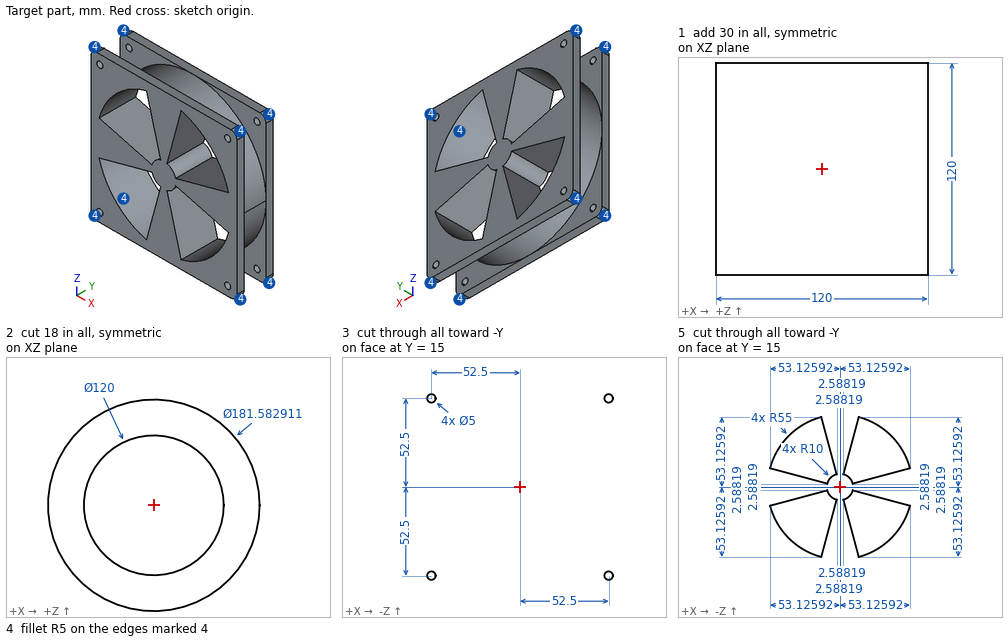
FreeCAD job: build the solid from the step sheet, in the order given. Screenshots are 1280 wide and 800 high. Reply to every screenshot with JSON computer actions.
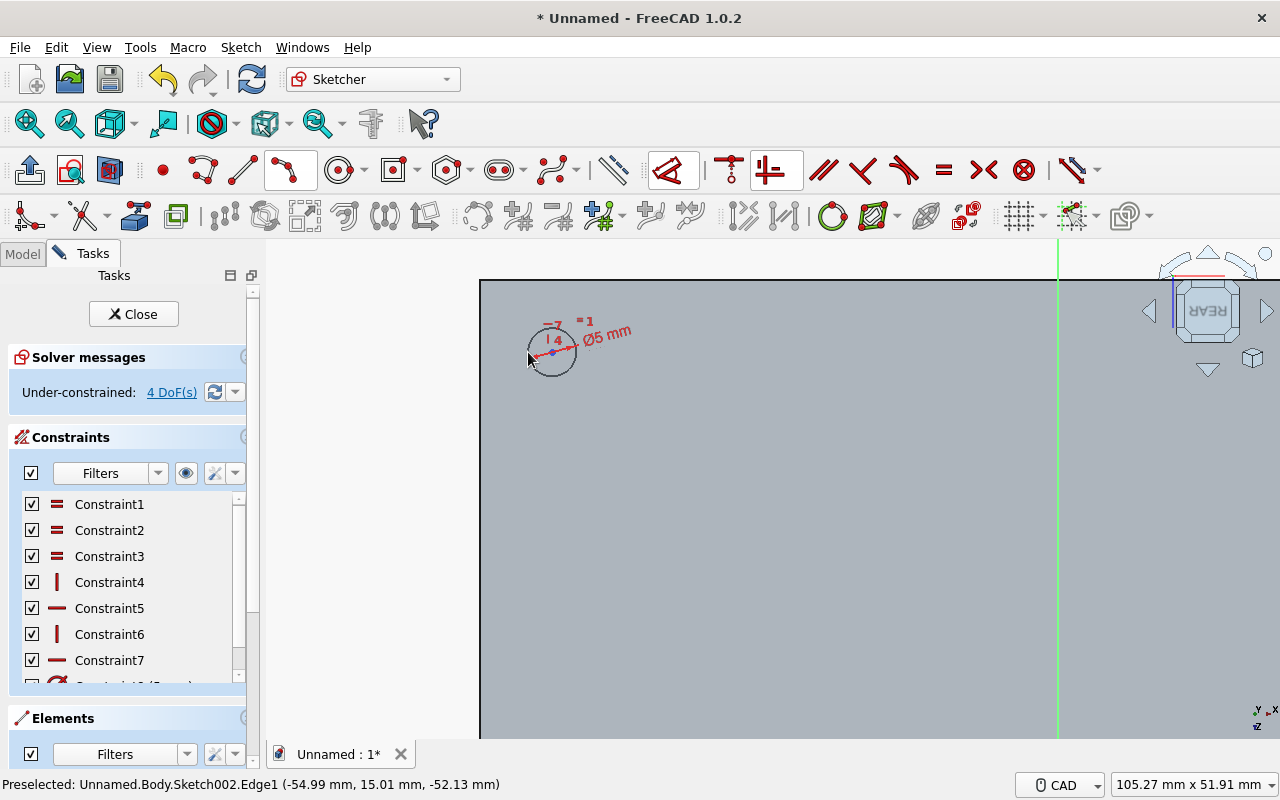
{"action": "left_click", "coordinate": [552, 352]}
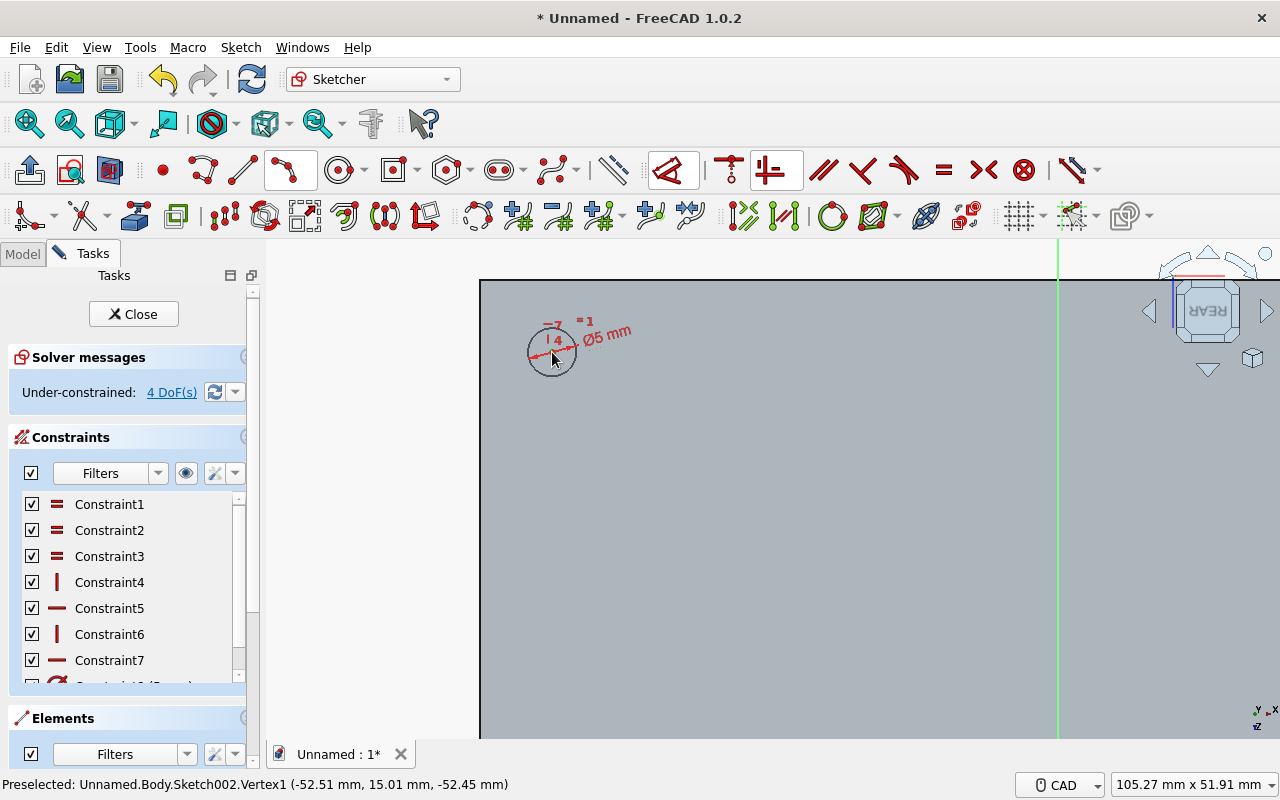
{"action": "key", "text": "l"}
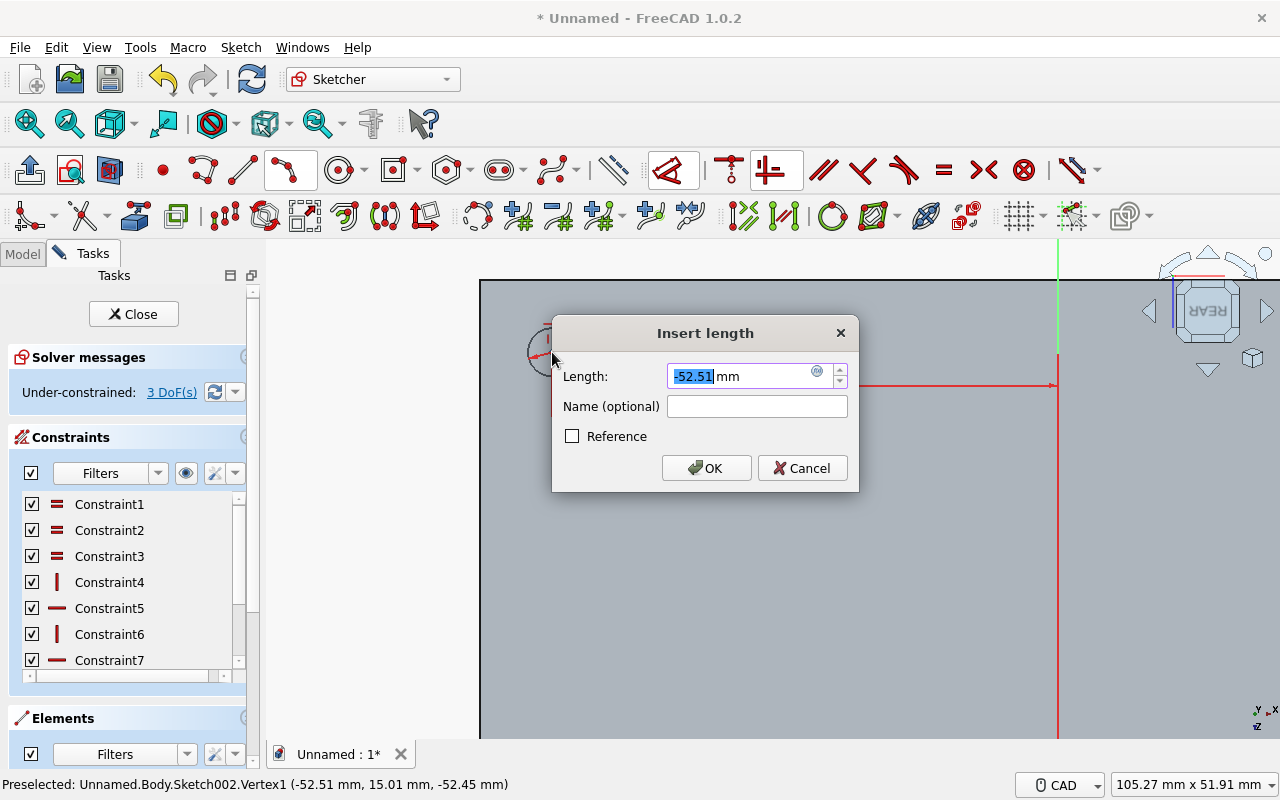
{"action": "type", "text": "-52.5"}
{"action": "key", "text": "Return"}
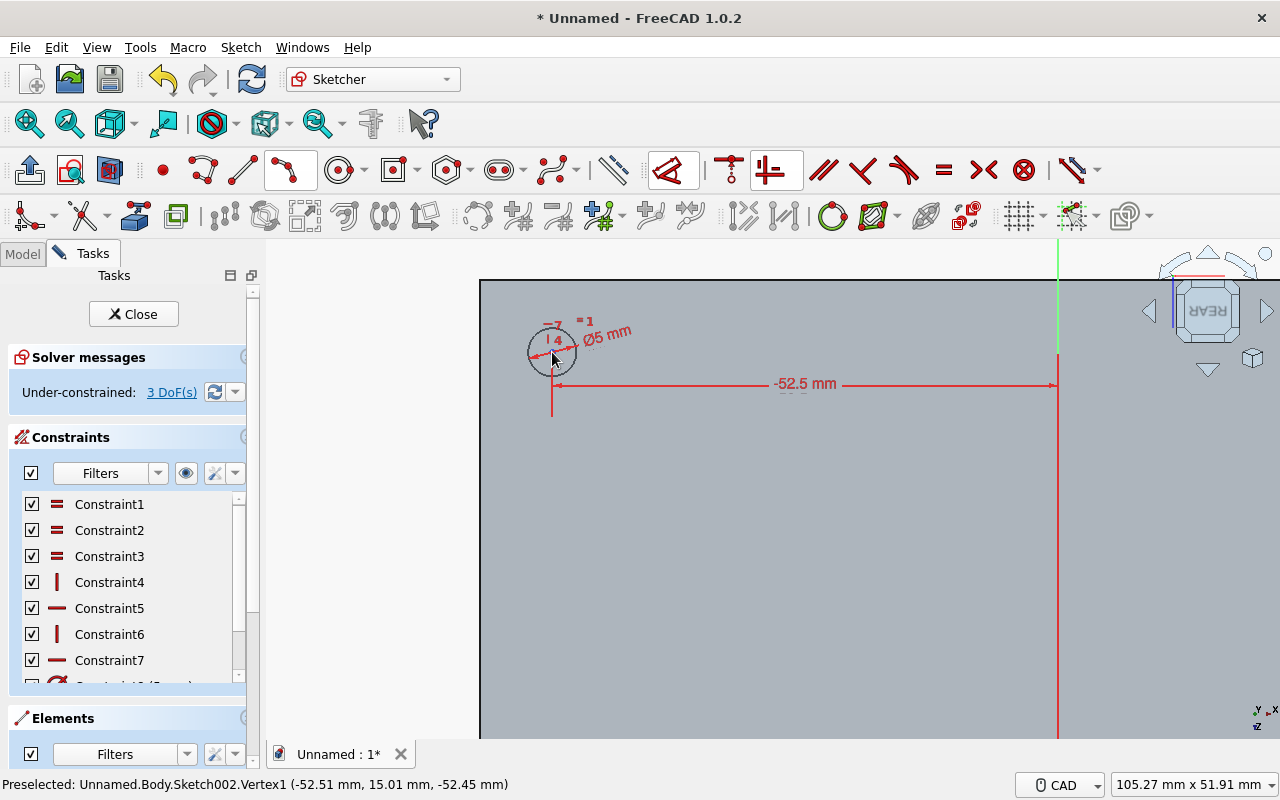
{"action": "left_click", "coordinate": [552, 352]}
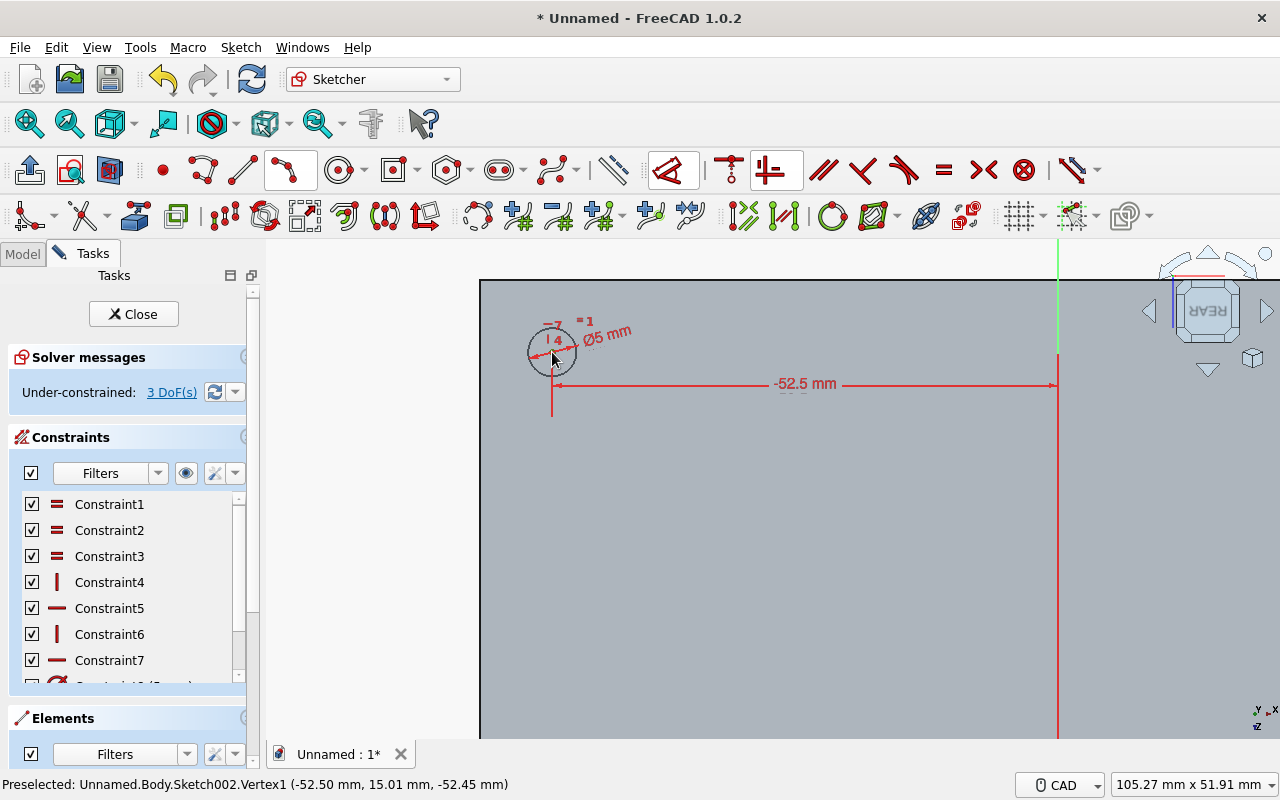
{"action": "left_click", "coordinate": [694, 170]}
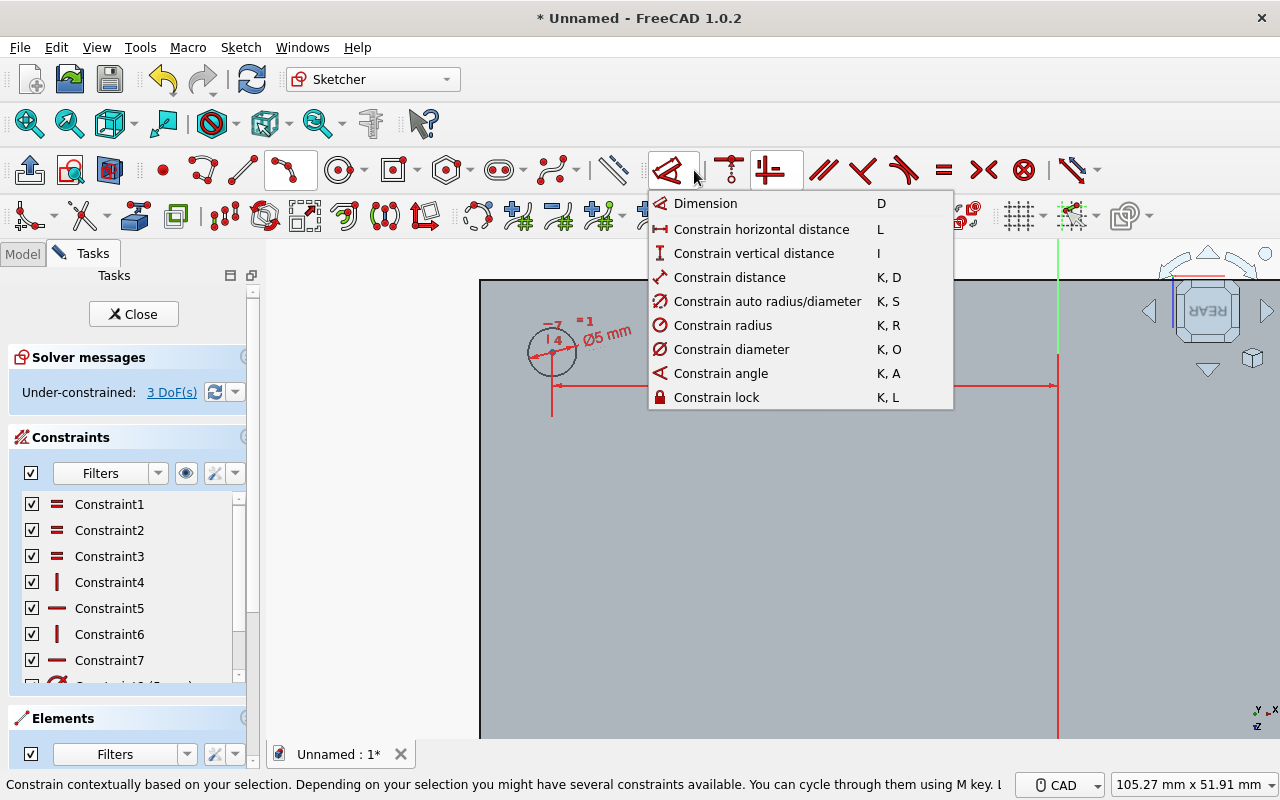
{"action": "left_click", "coordinate": [801, 253]}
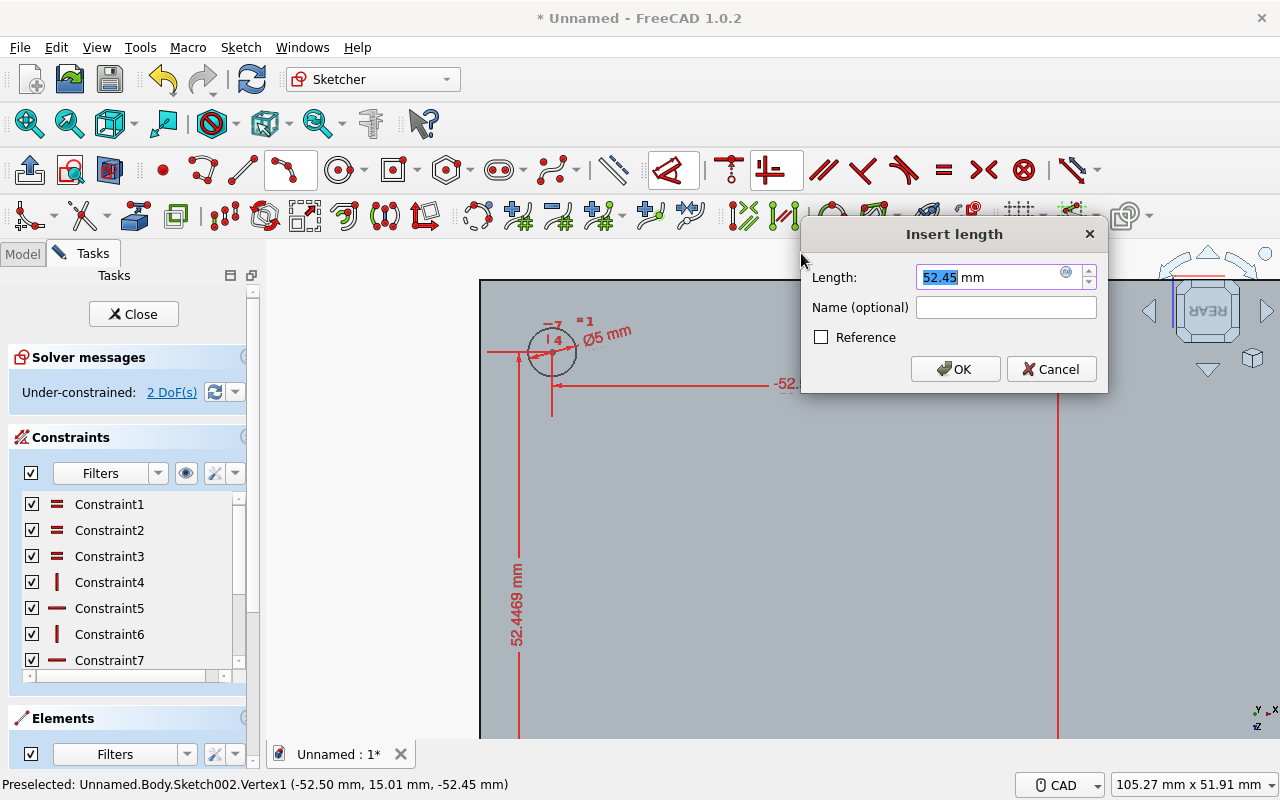
{"action": "type", "text": "52.5"}
{"action": "key", "text": "Return"}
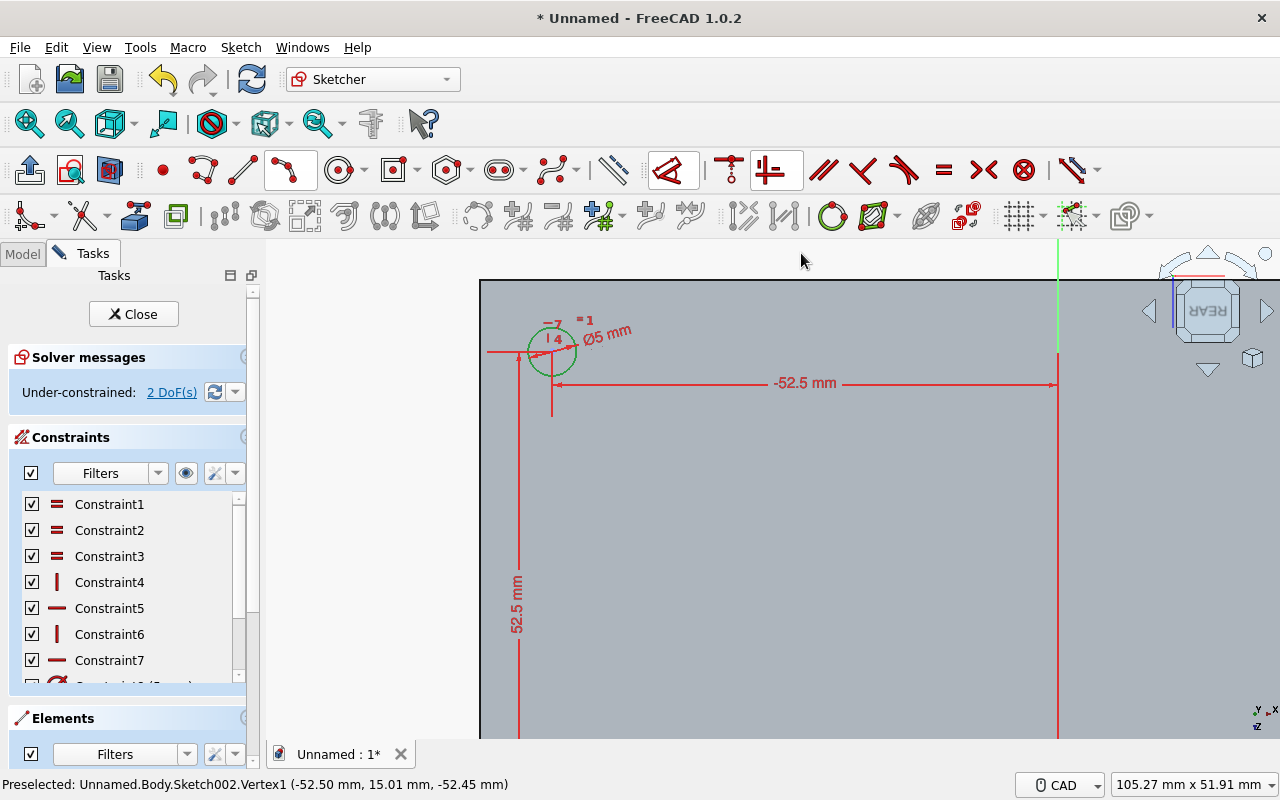
{"action": "scroll", "coordinate": [552, 330], "scroll_direction": "down", "scroll_amount": 6}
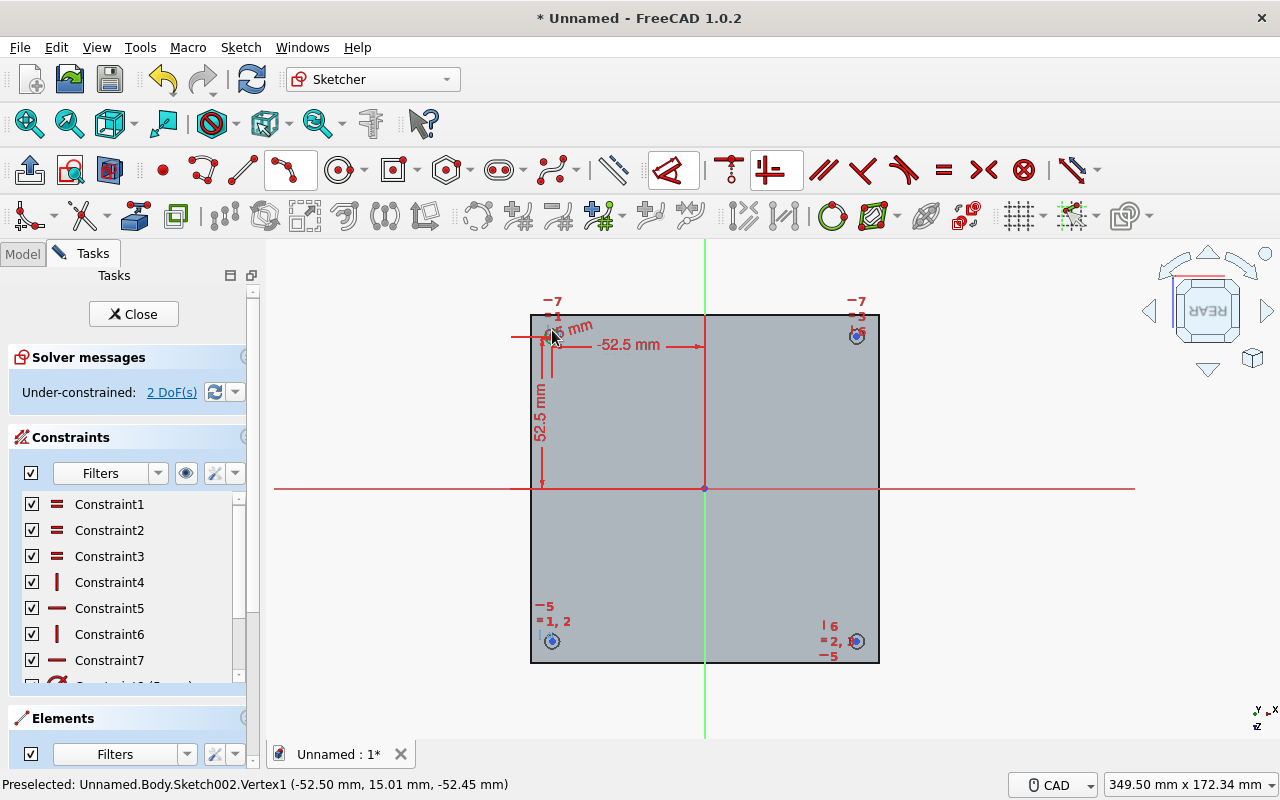
{"action": "left_click", "coordinate": [552, 642]}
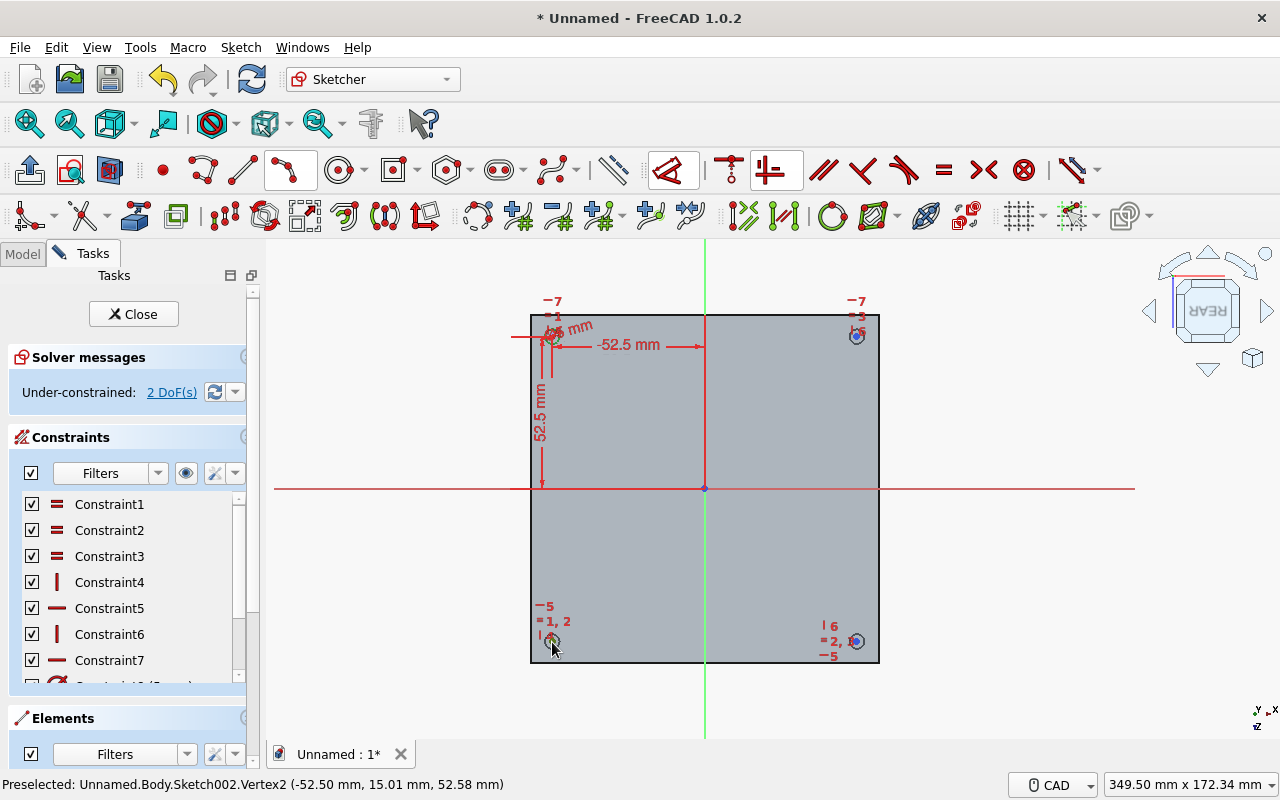
{"action": "left_click", "coordinate": [694, 170]}